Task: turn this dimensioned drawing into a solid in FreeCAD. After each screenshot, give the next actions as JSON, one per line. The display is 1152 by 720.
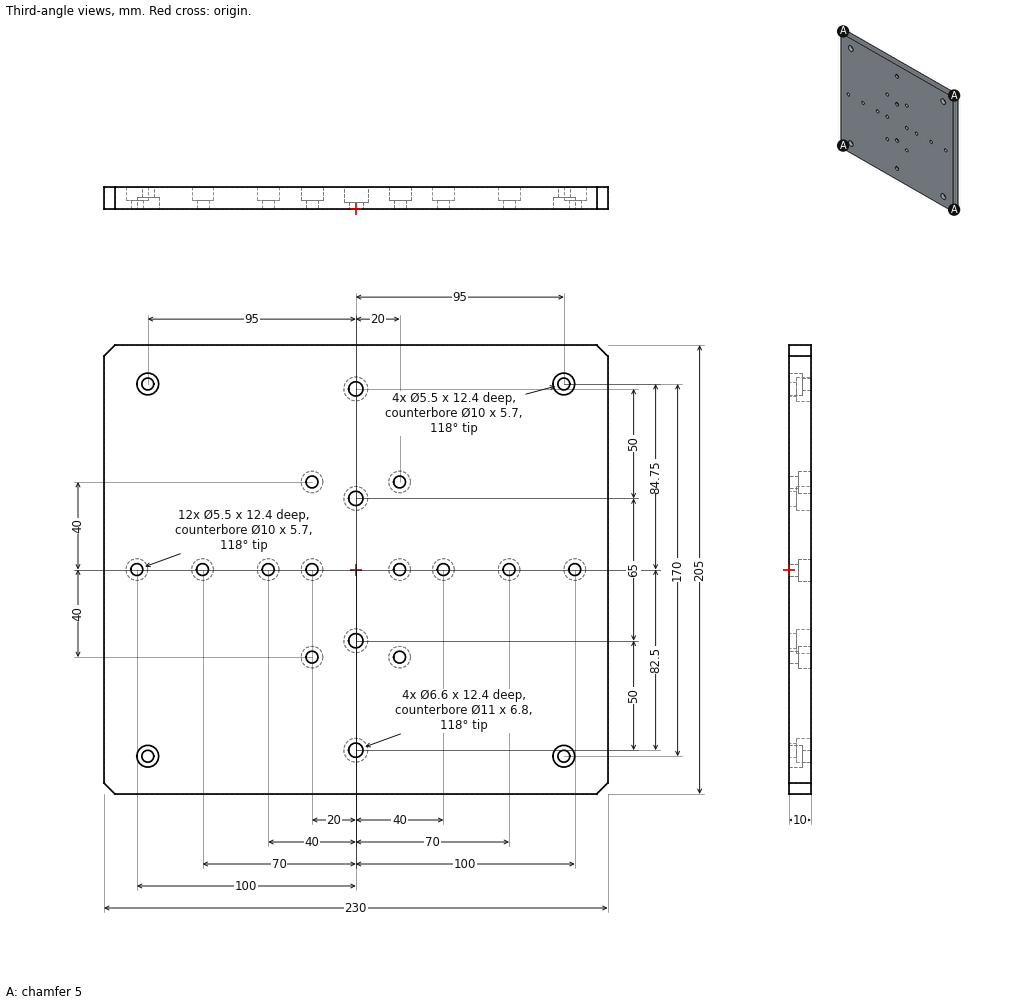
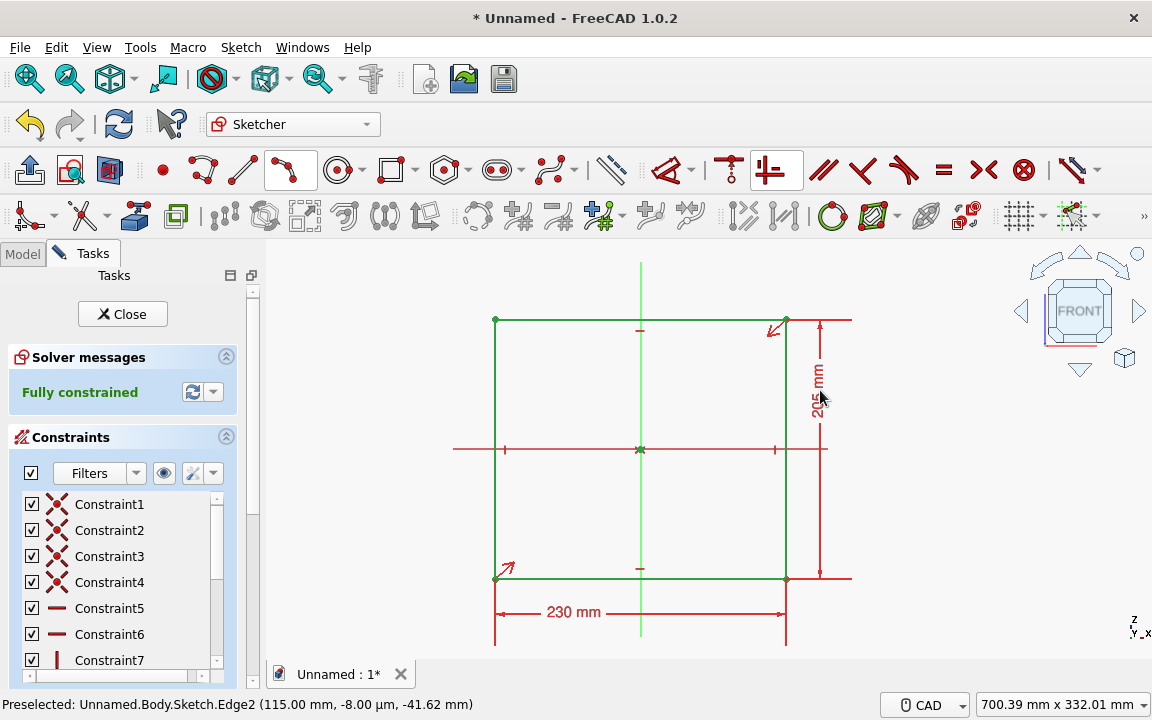
{"action": "left_click", "coordinate": [123, 314]}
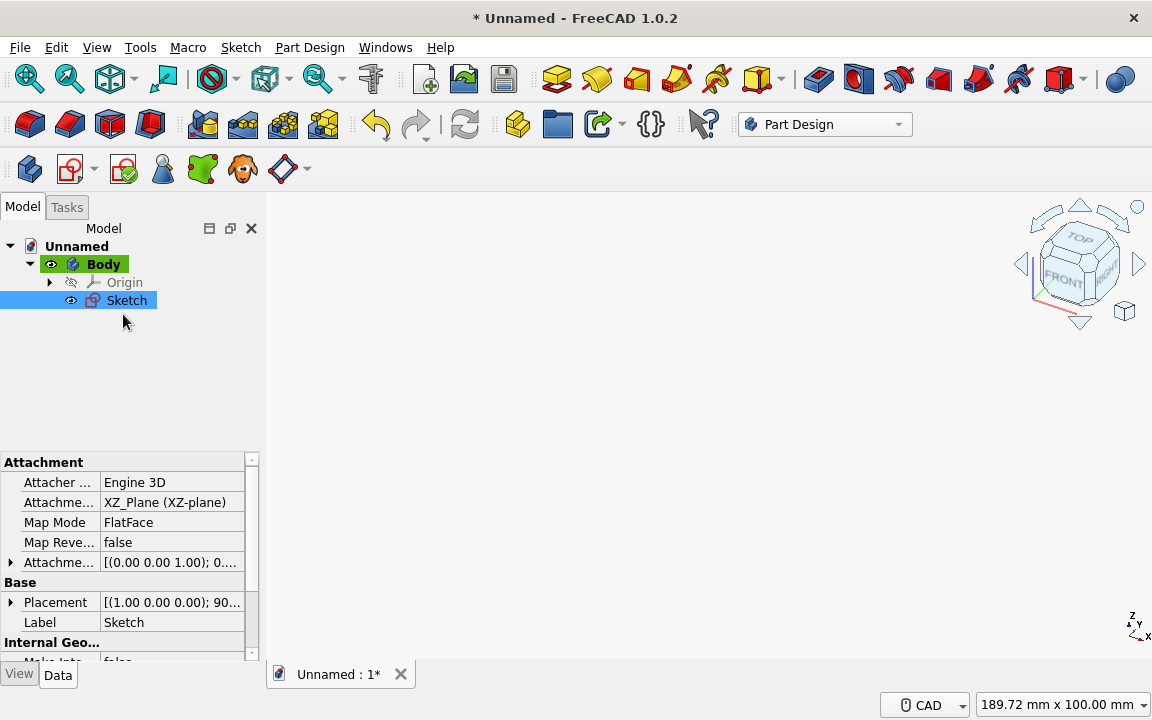
{"action": "left_click", "coordinate": [558, 80]}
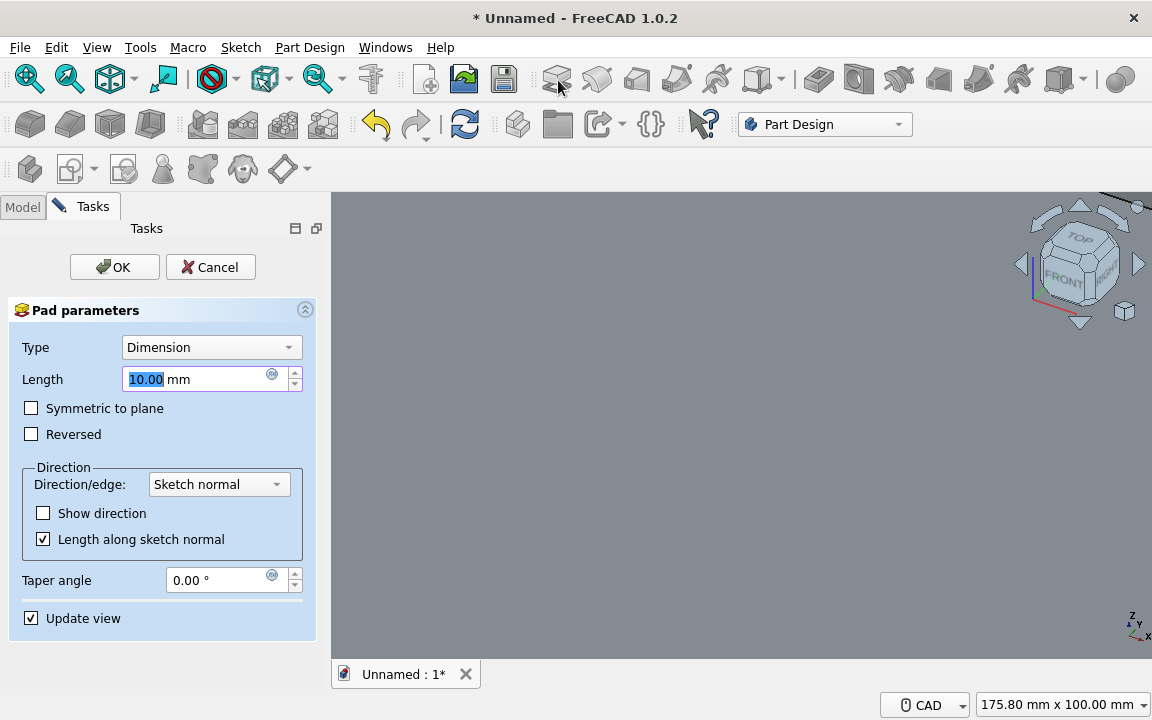
{"action": "type", "text": "10"}
{"action": "key", "text": "Tab"}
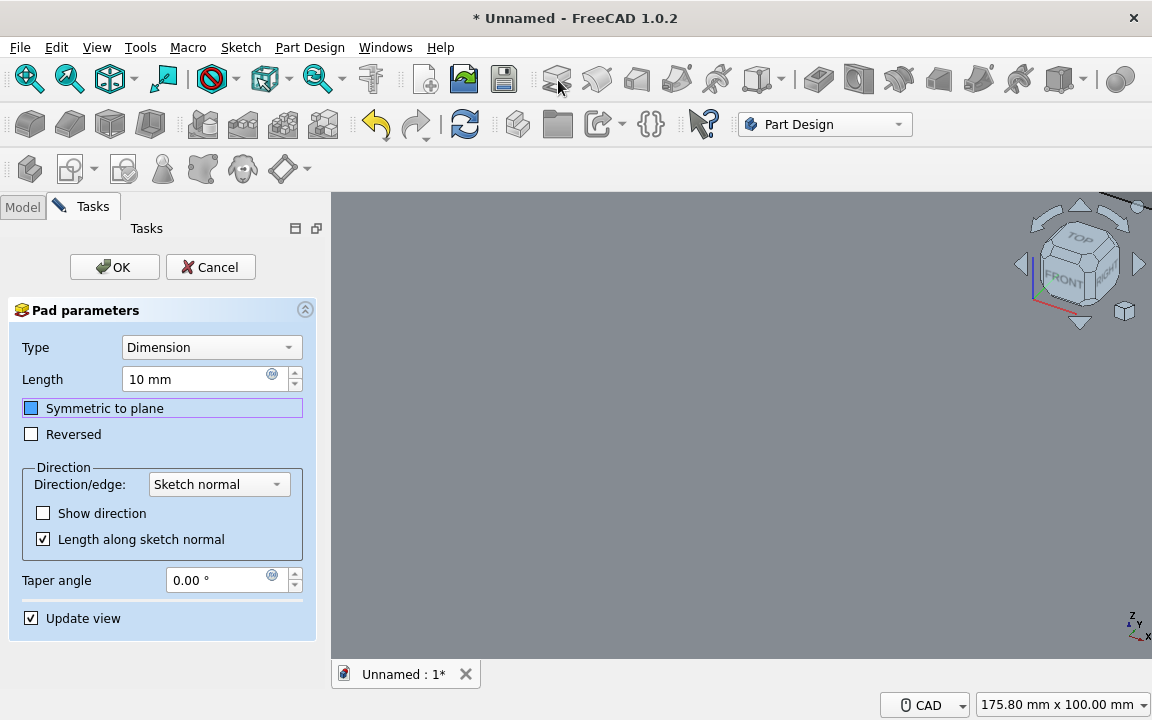
{"action": "left_click", "coordinate": [30, 434]}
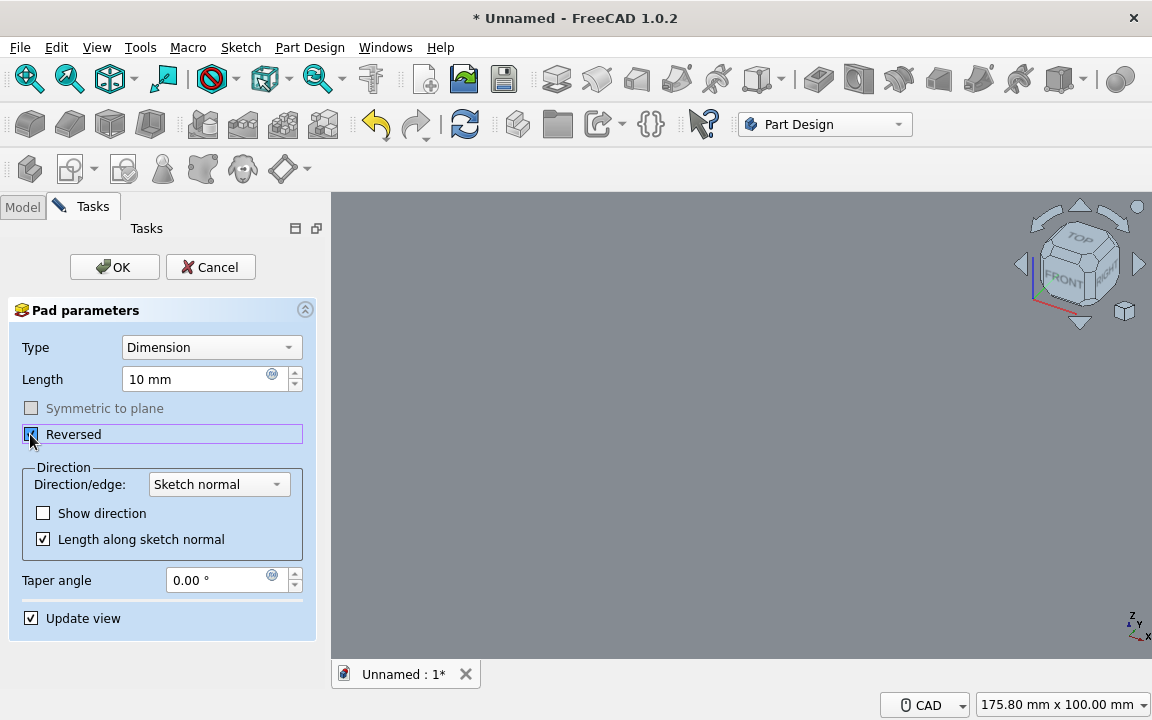
{"action": "left_click", "coordinate": [115, 267]}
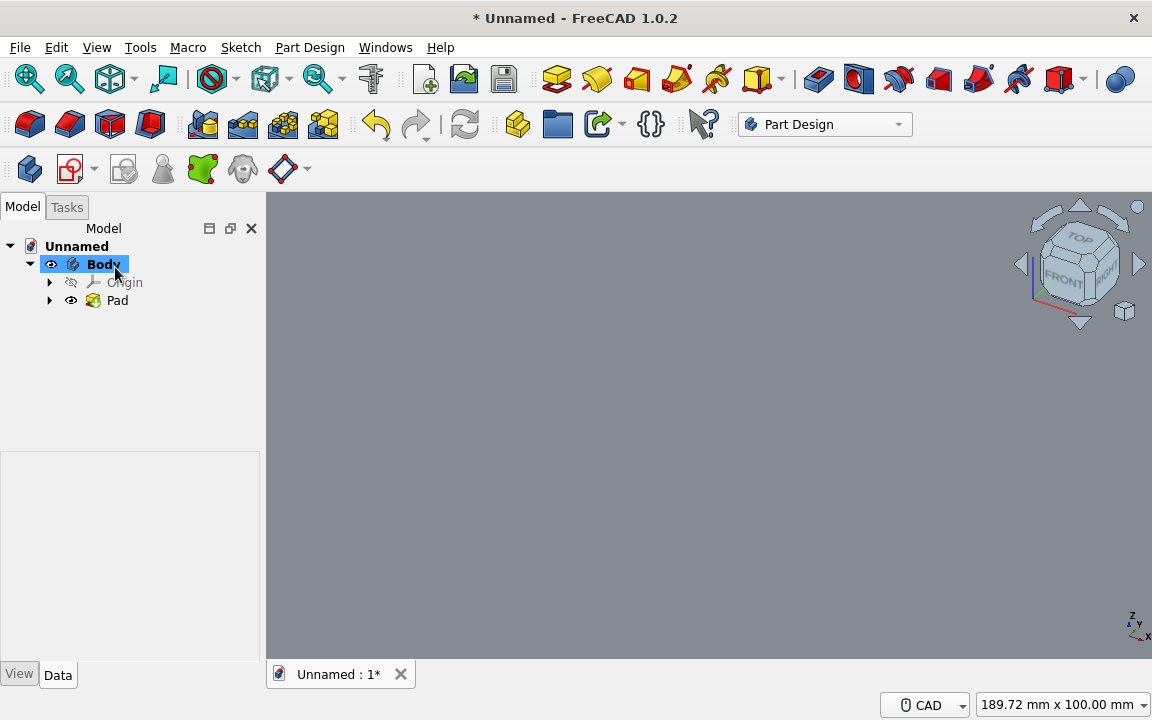
{"action": "left_click", "coordinate": [30, 80]}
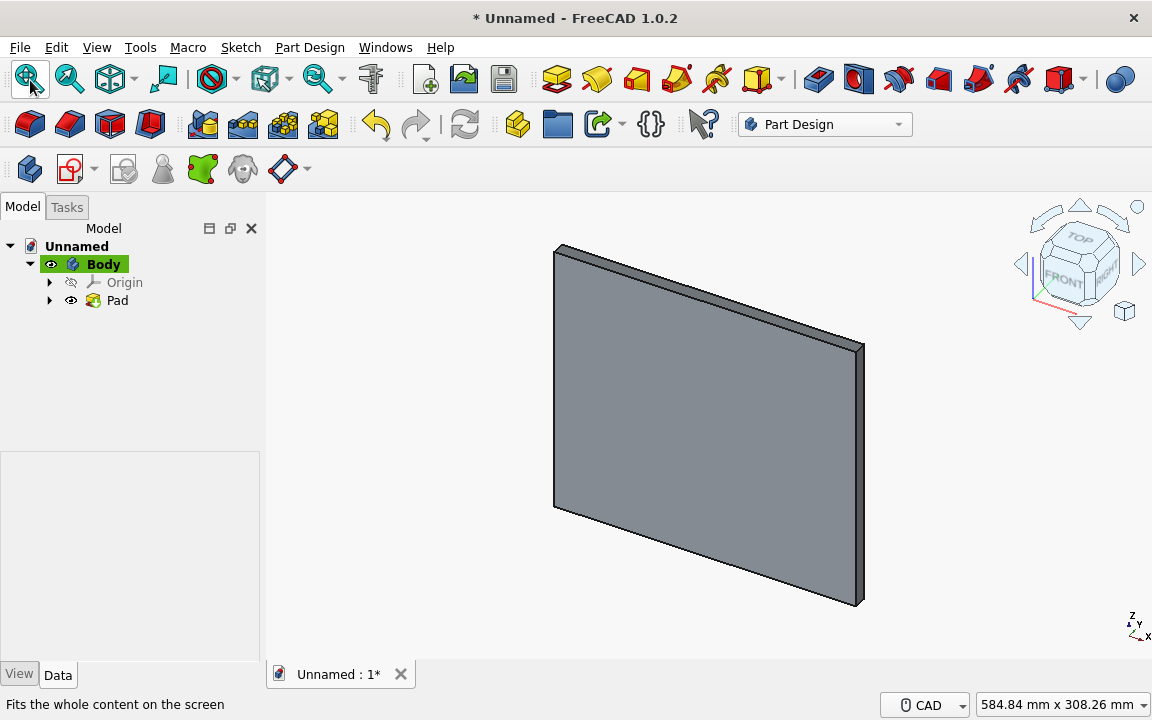
{"action": "left_click", "coordinate": [70, 170]}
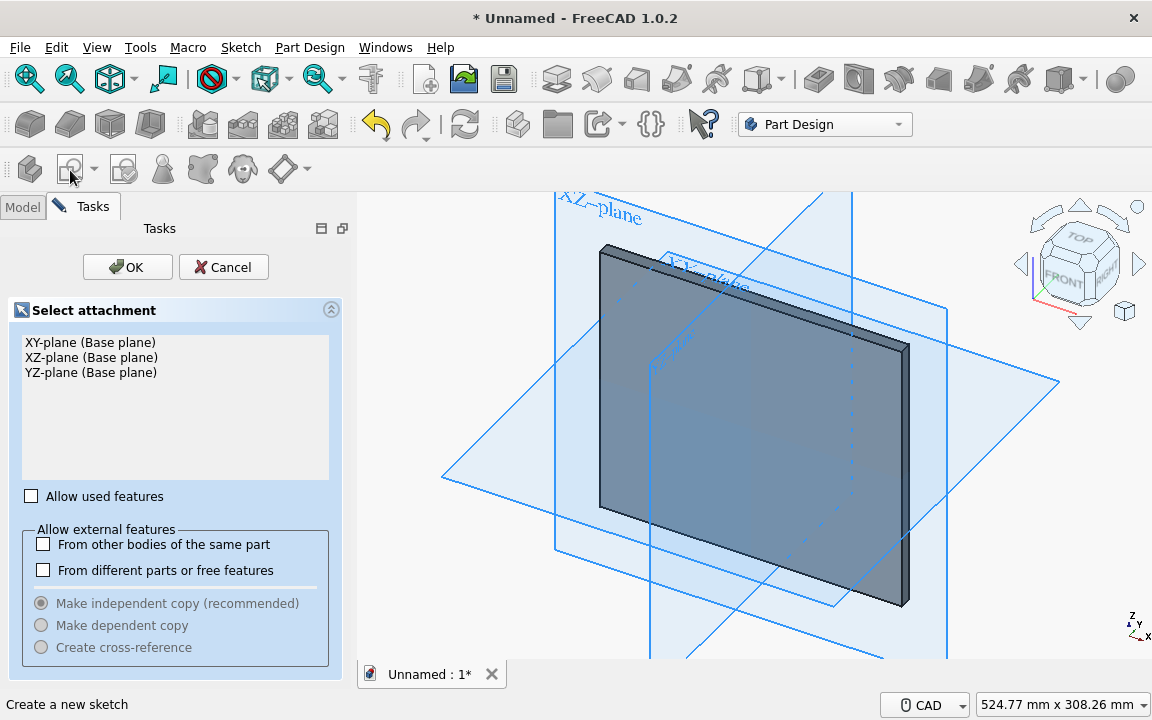
{"action": "left_click", "coordinate": [82, 358]}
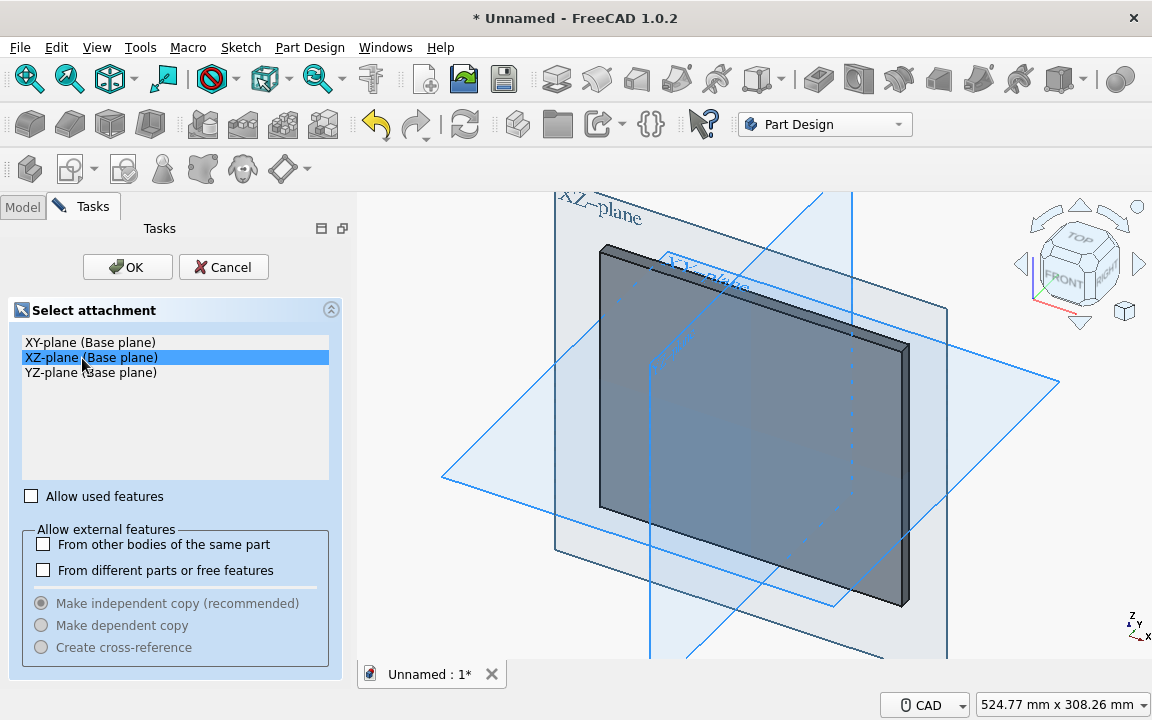
{"action": "left_click", "coordinate": [128, 267]}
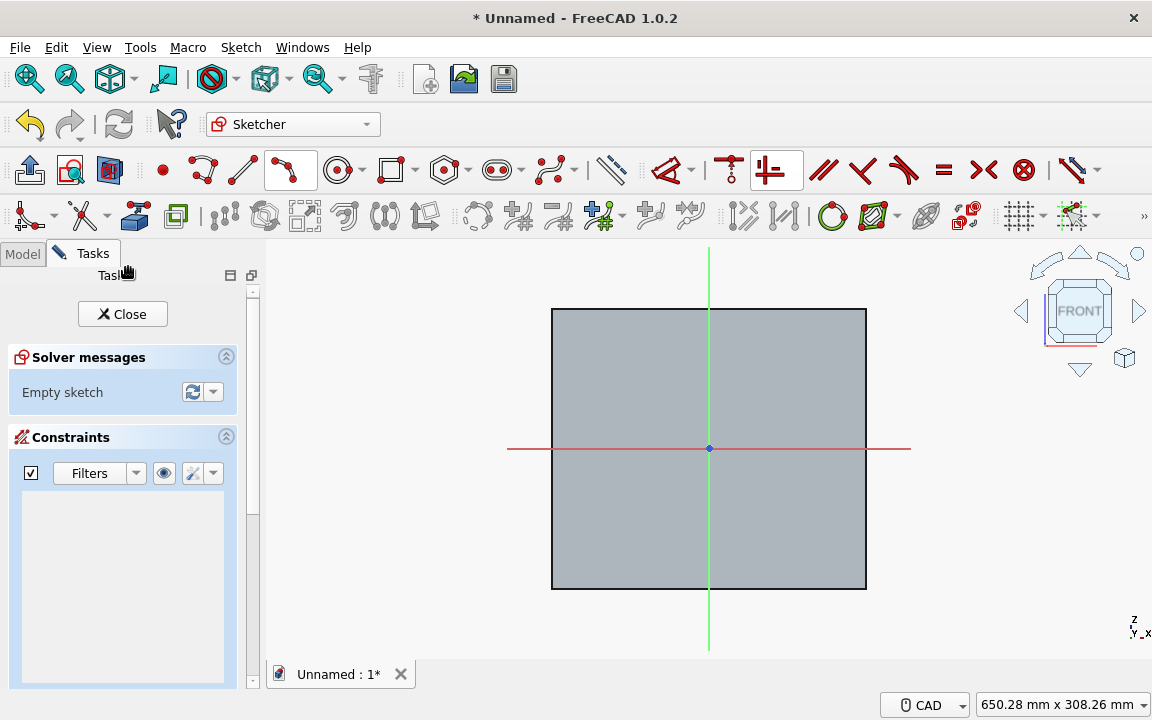
{"action": "left_click", "coordinate": [338, 170]}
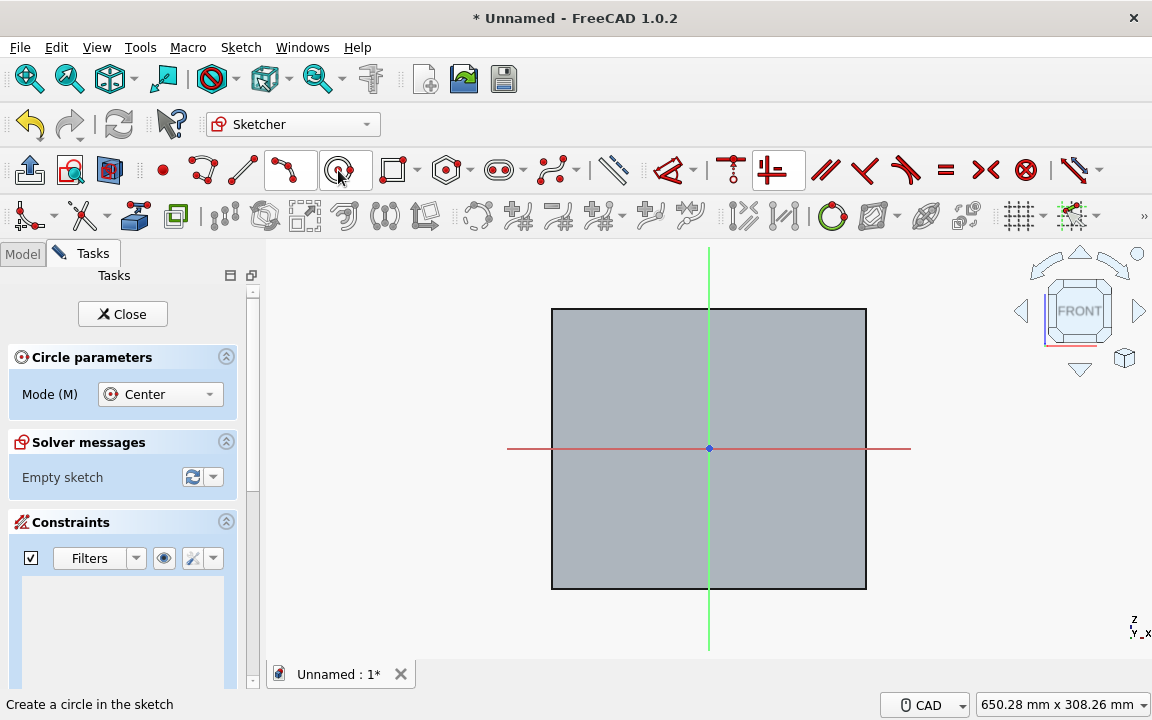
{"action": "scroll", "coordinate": [838, 334], "scroll_direction": "up", "scroll_amount": 10}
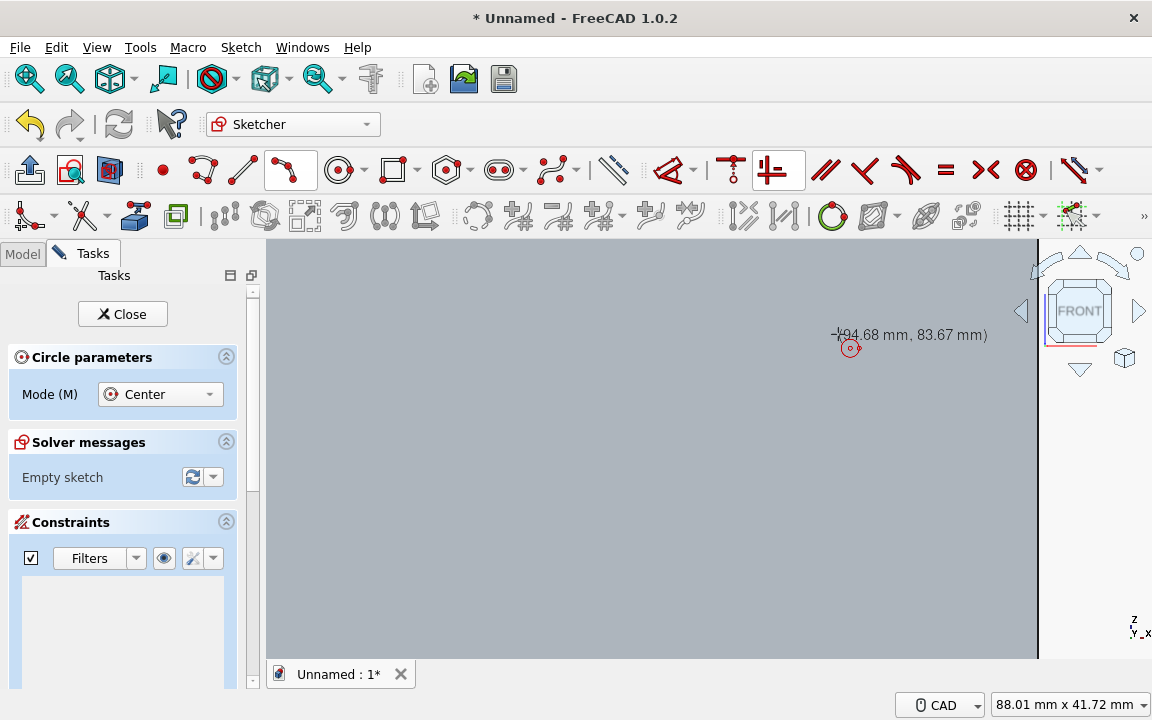
{"action": "scroll", "coordinate": [759, 334], "scroll_direction": "down", "scroll_amount": 10}